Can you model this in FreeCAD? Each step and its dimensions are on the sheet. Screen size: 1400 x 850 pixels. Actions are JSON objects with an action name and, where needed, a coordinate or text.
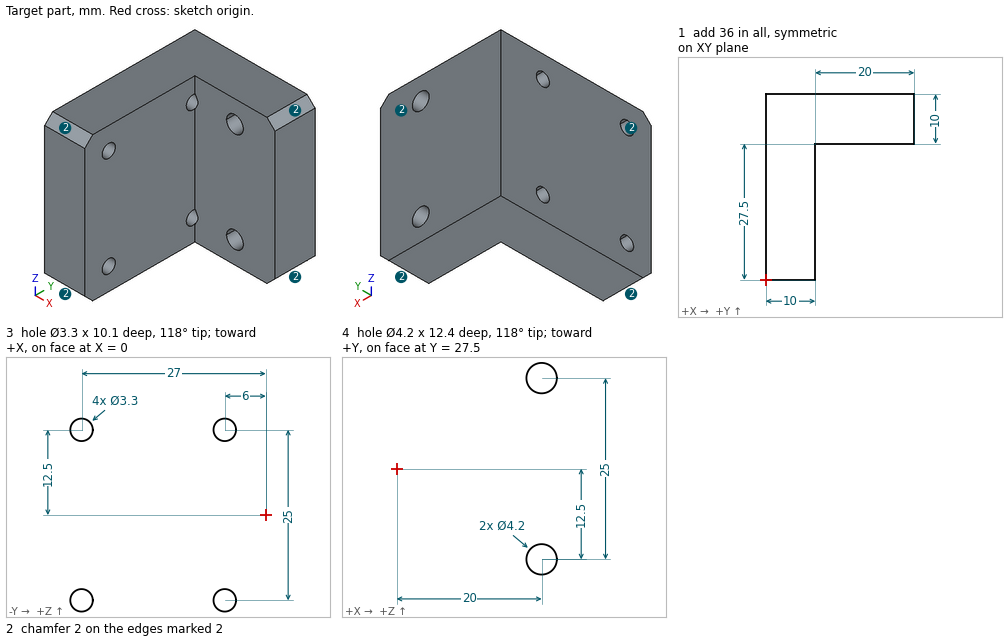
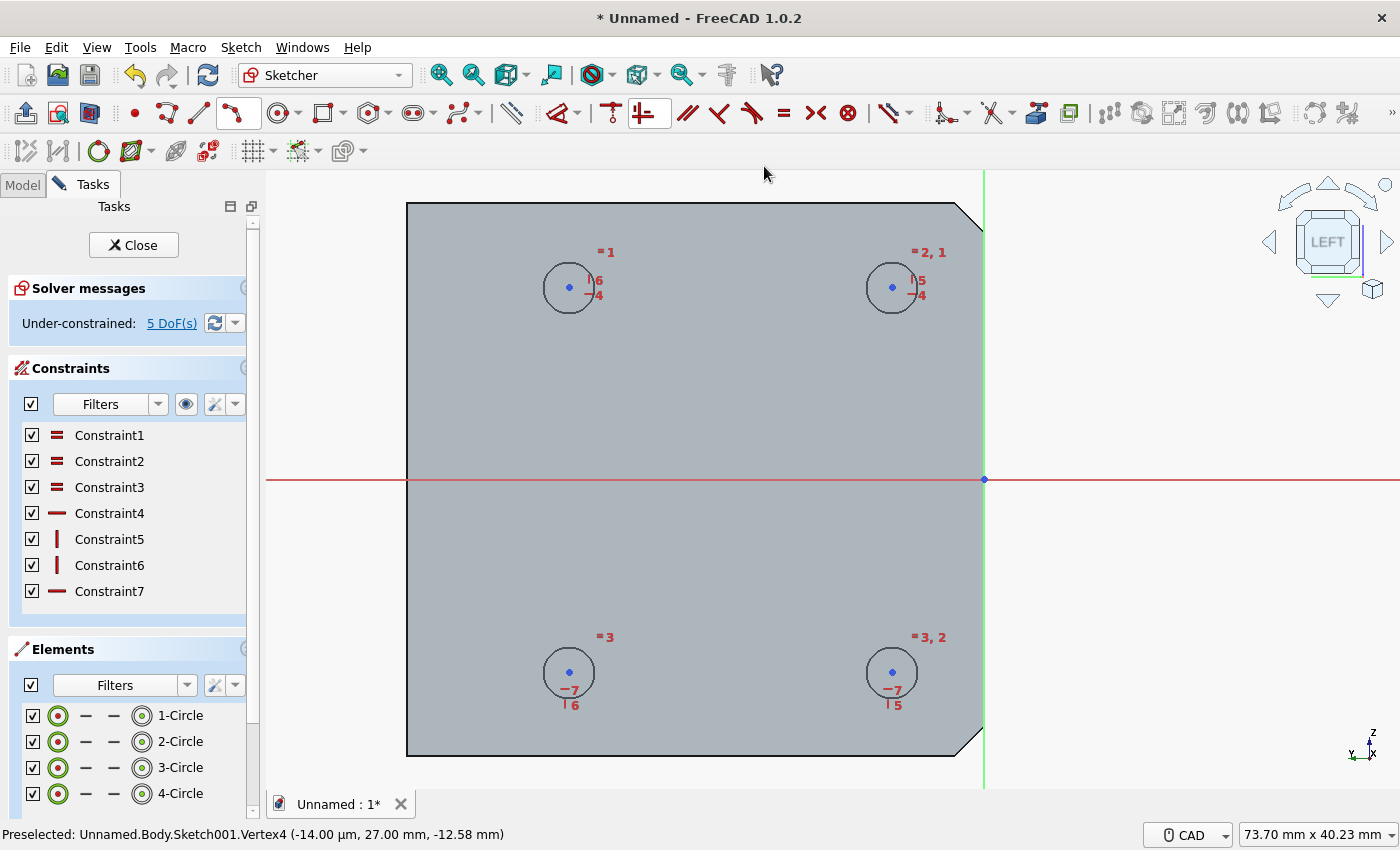
{"action": "key", "text": "d"}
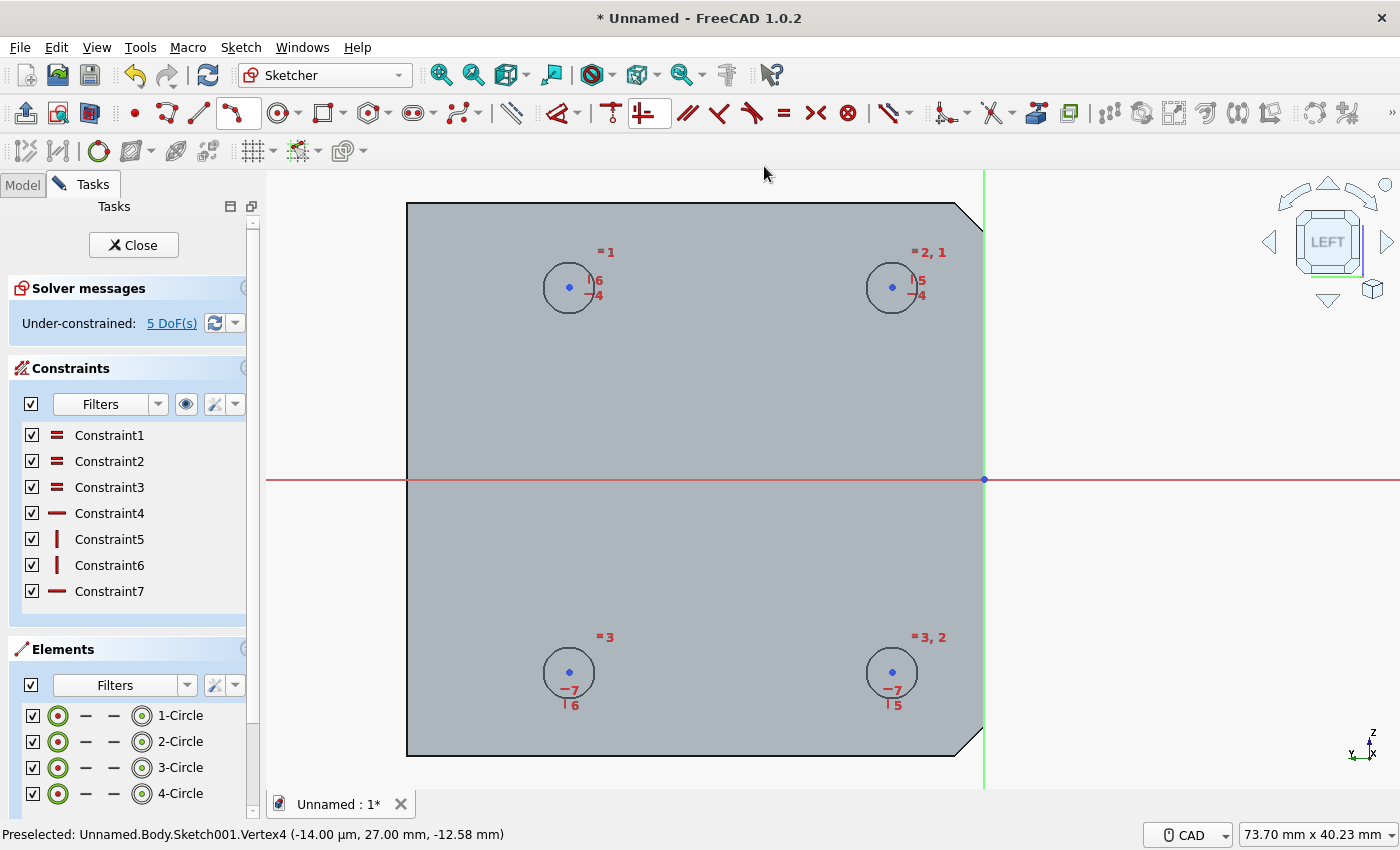
{"action": "left_click", "coordinate": [587, 270]}
{"action": "left_click", "coordinate": [610, 247]}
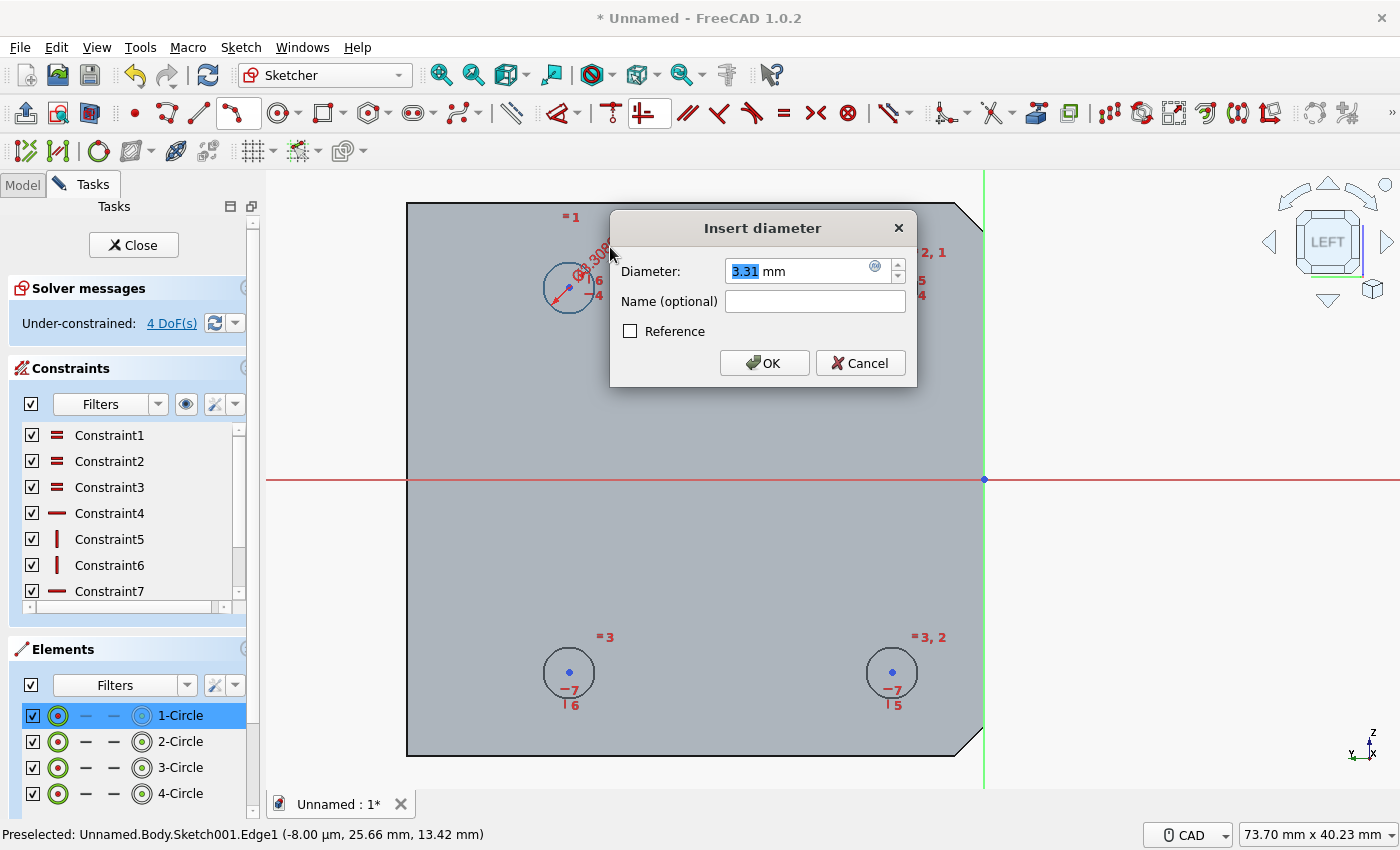
{"action": "type", "text": "3.3"}
{"action": "key", "text": "Return"}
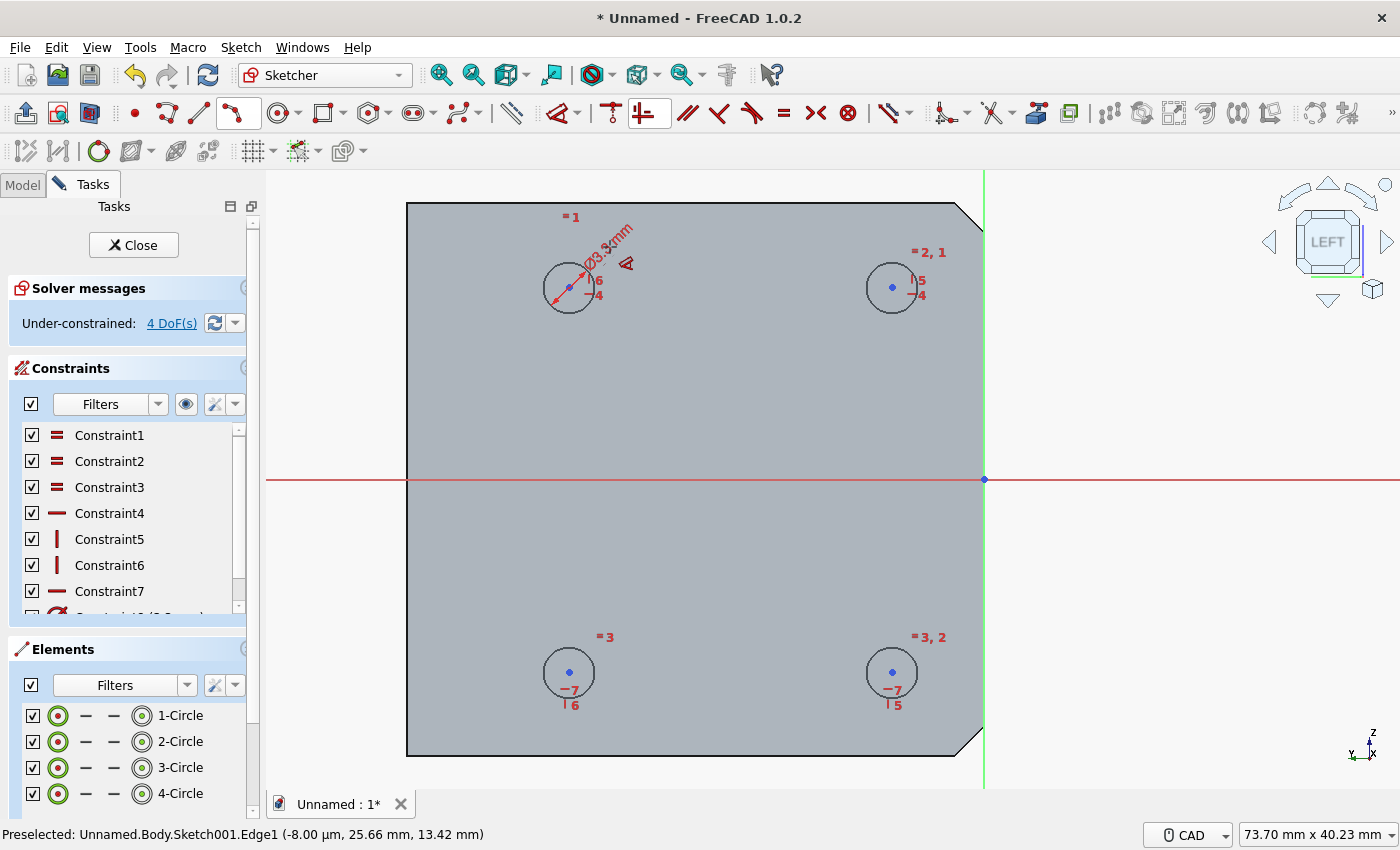
{"action": "left_click", "coordinate": [892, 288]}
{"action": "left_click", "coordinate": [938, 254]}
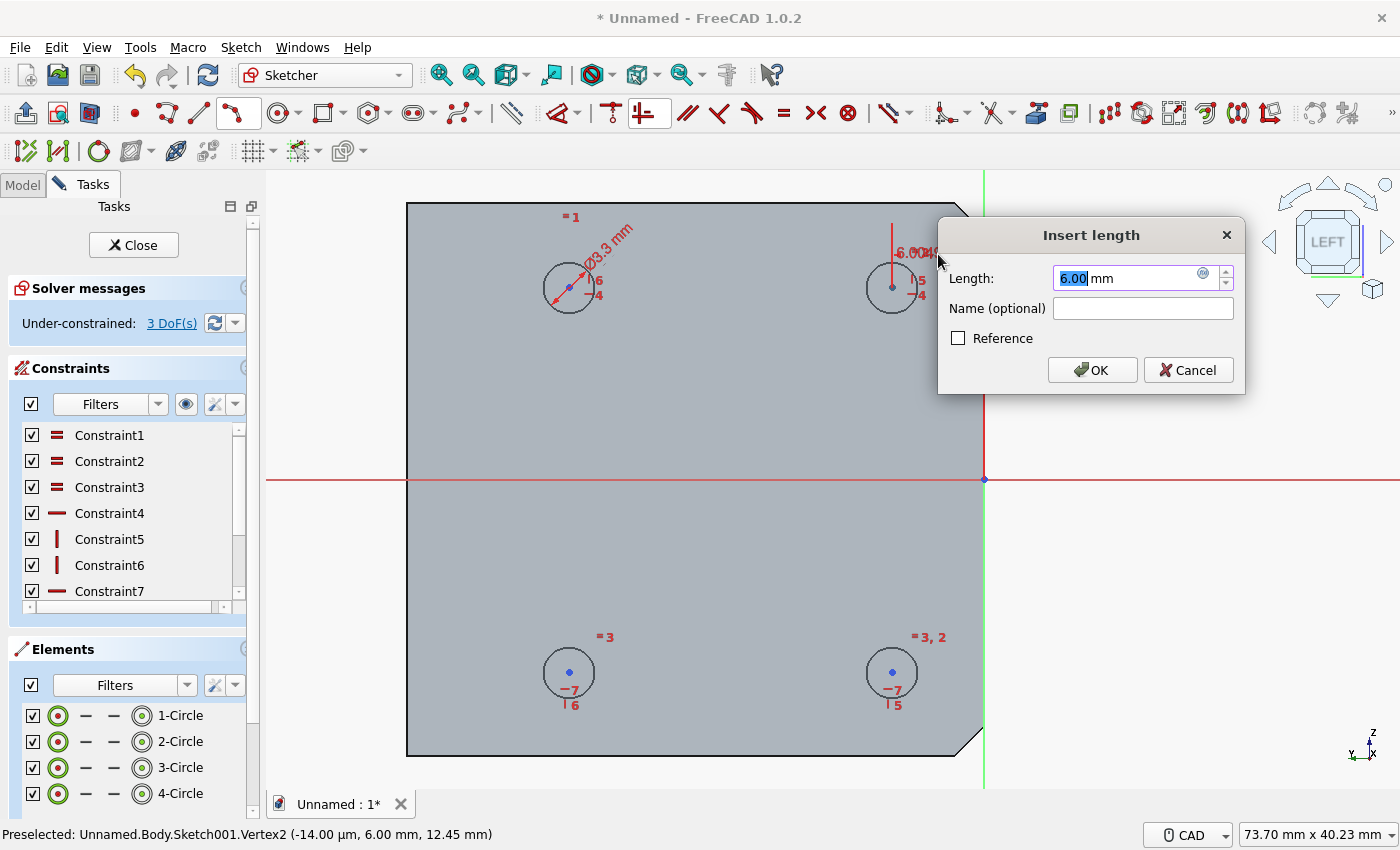
{"action": "type", "text": "6"}
{"action": "key", "text": "Return"}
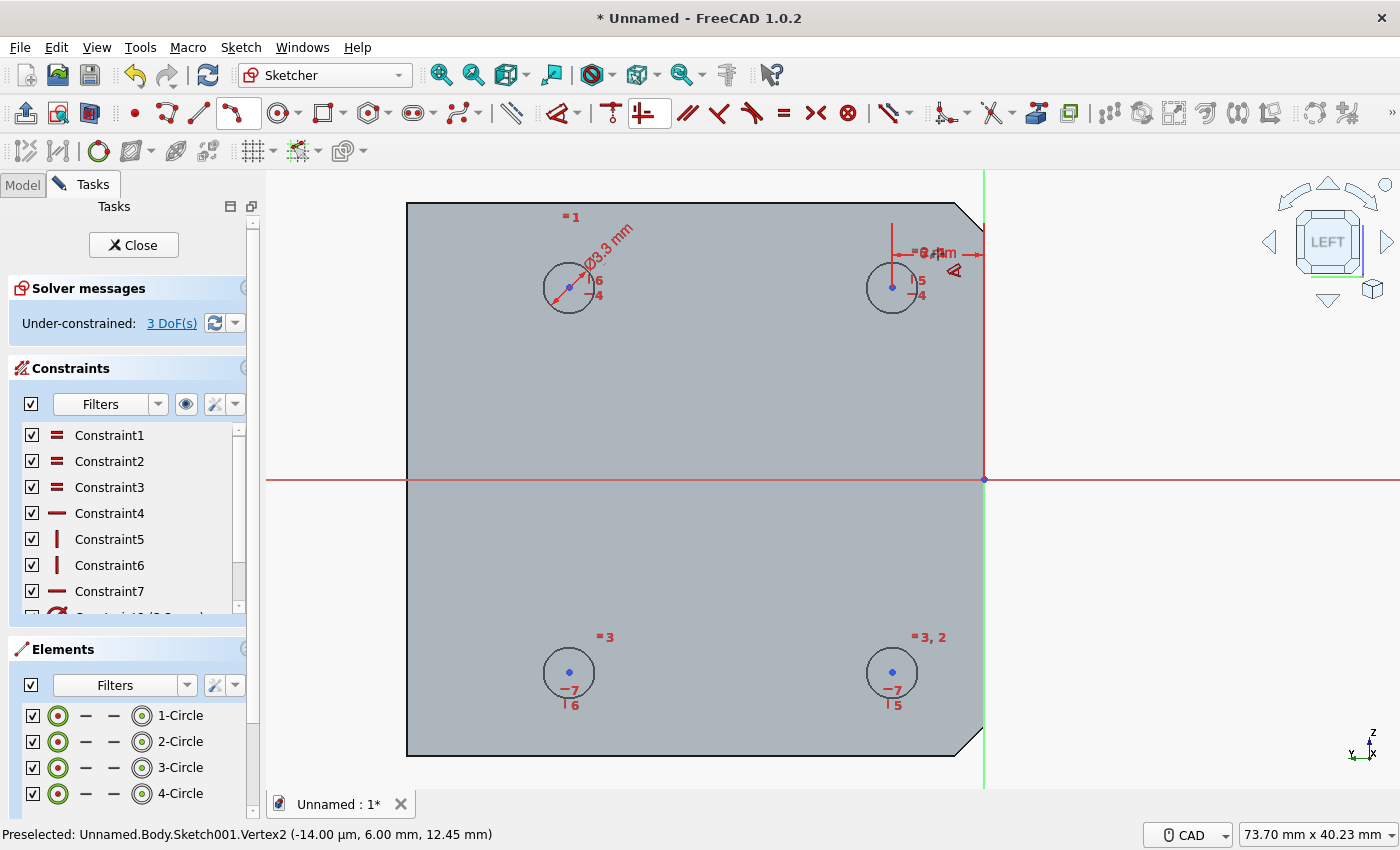
{"action": "left_click", "coordinate": [569, 288]}
{"action": "left_click", "coordinate": [777, 254]}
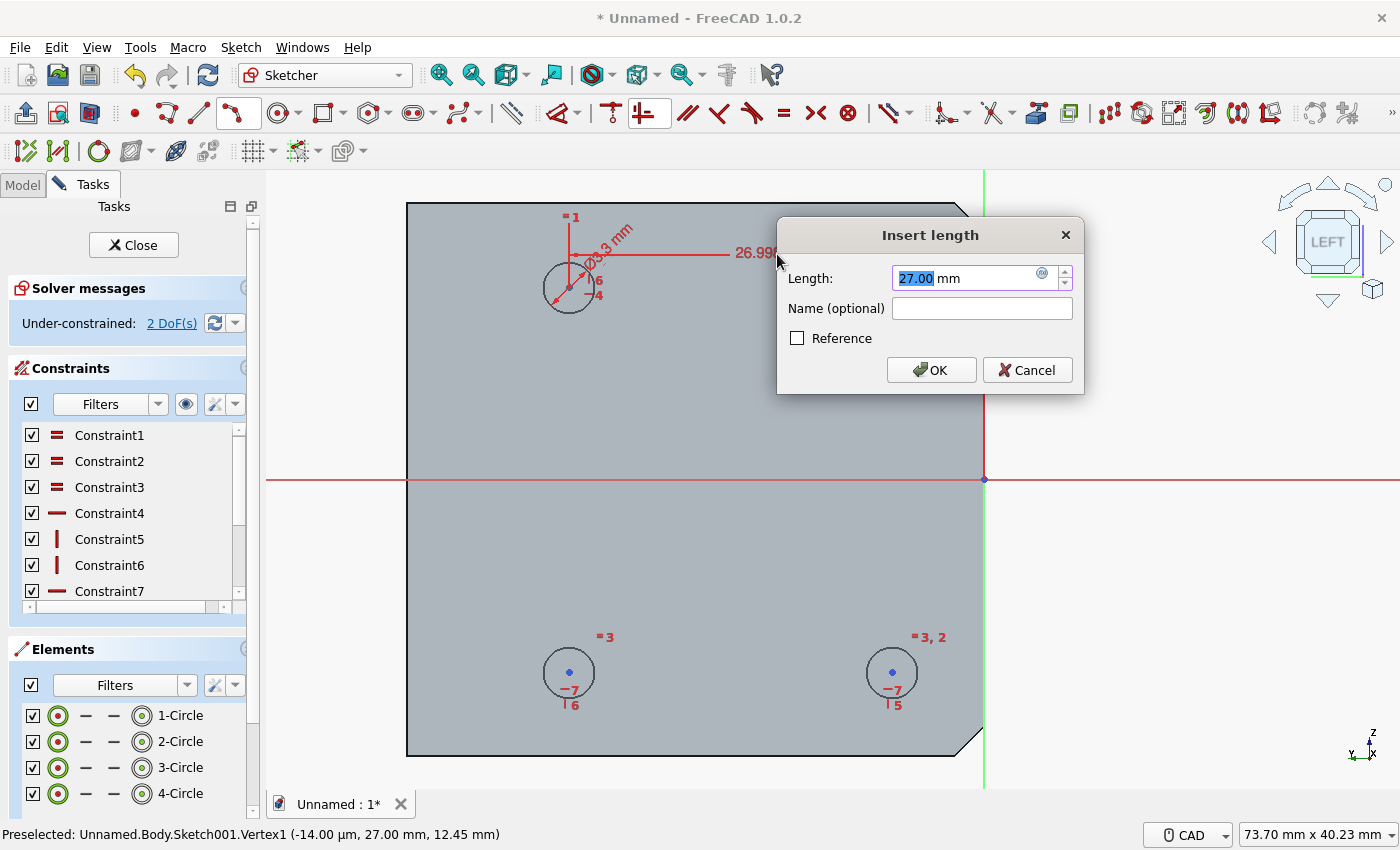
{"action": "type", "text": "27"}
{"action": "key", "text": "Return"}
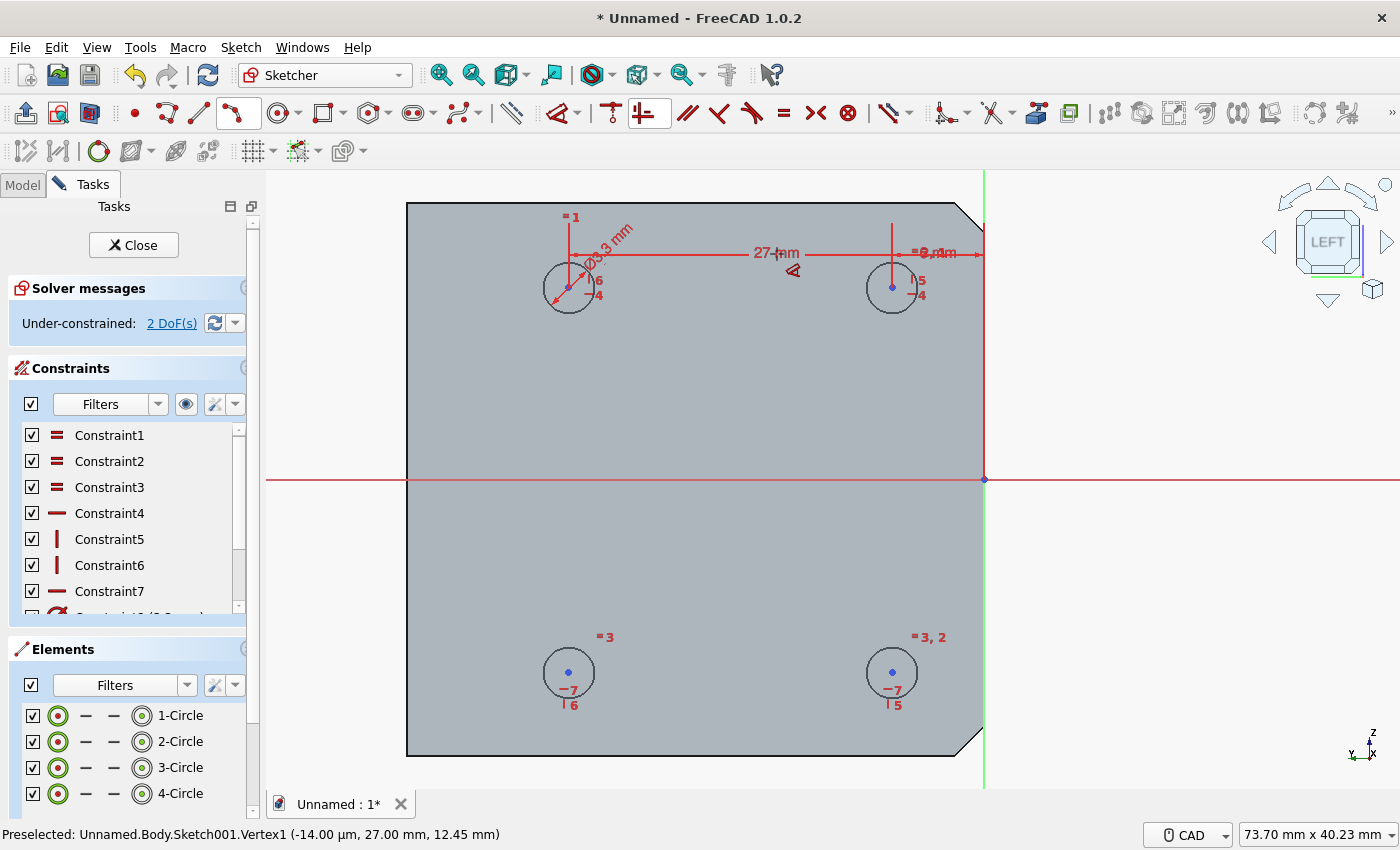
{"action": "left_click", "coordinate": [892, 288]}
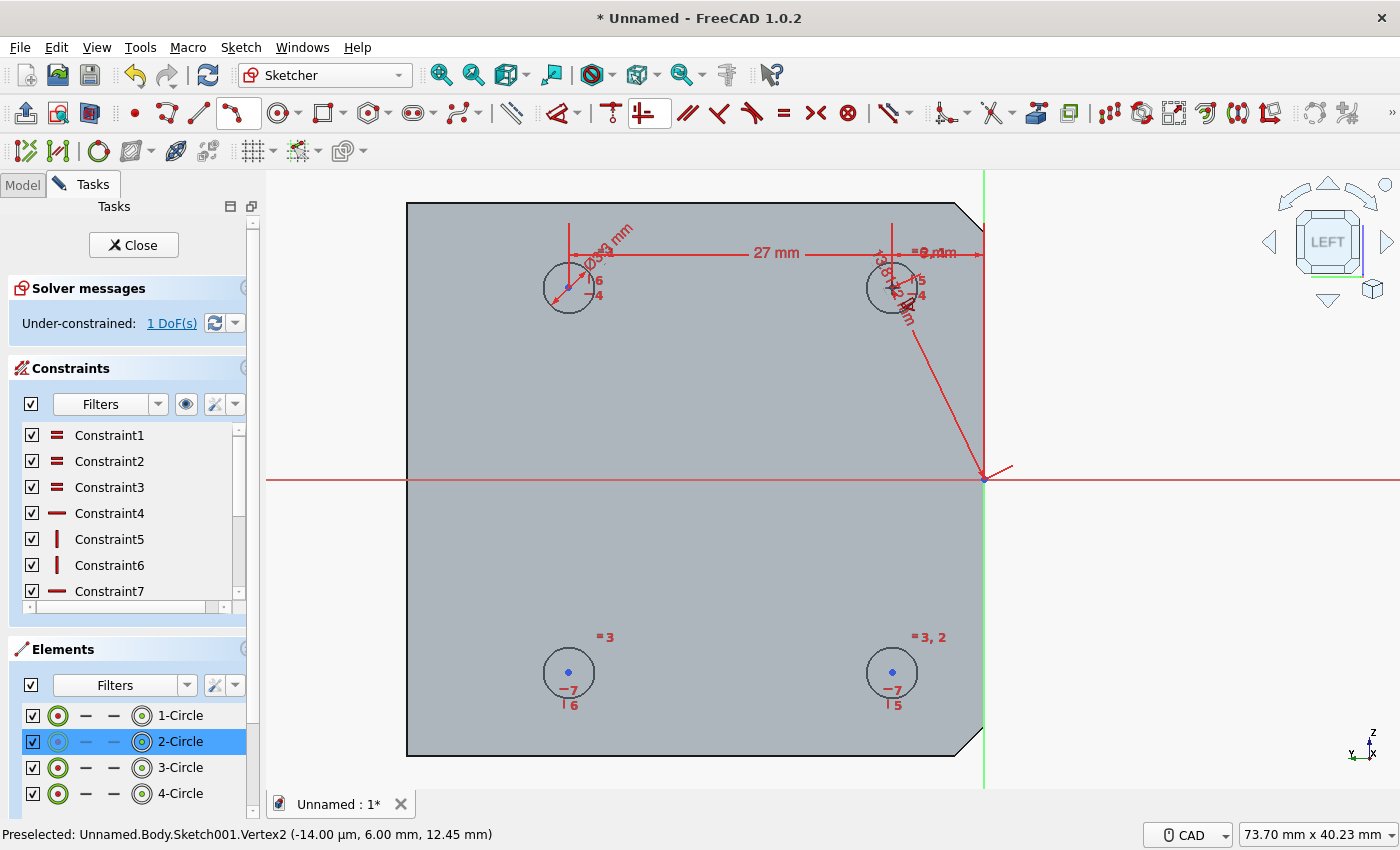
{"action": "left_click", "coordinate": [892, 673]}
{"action": "left_click", "coordinate": [926, 392]}